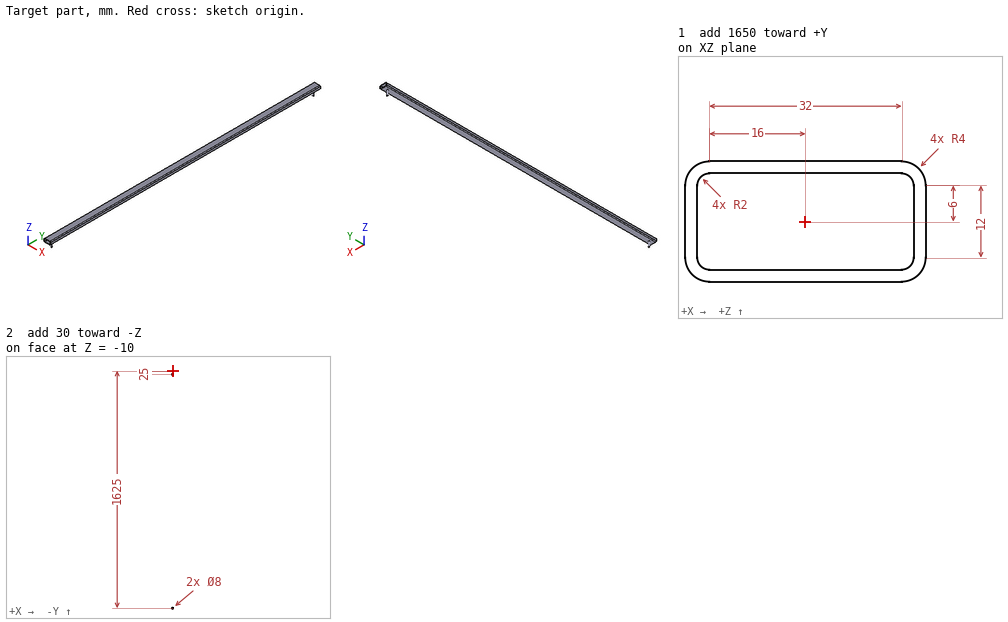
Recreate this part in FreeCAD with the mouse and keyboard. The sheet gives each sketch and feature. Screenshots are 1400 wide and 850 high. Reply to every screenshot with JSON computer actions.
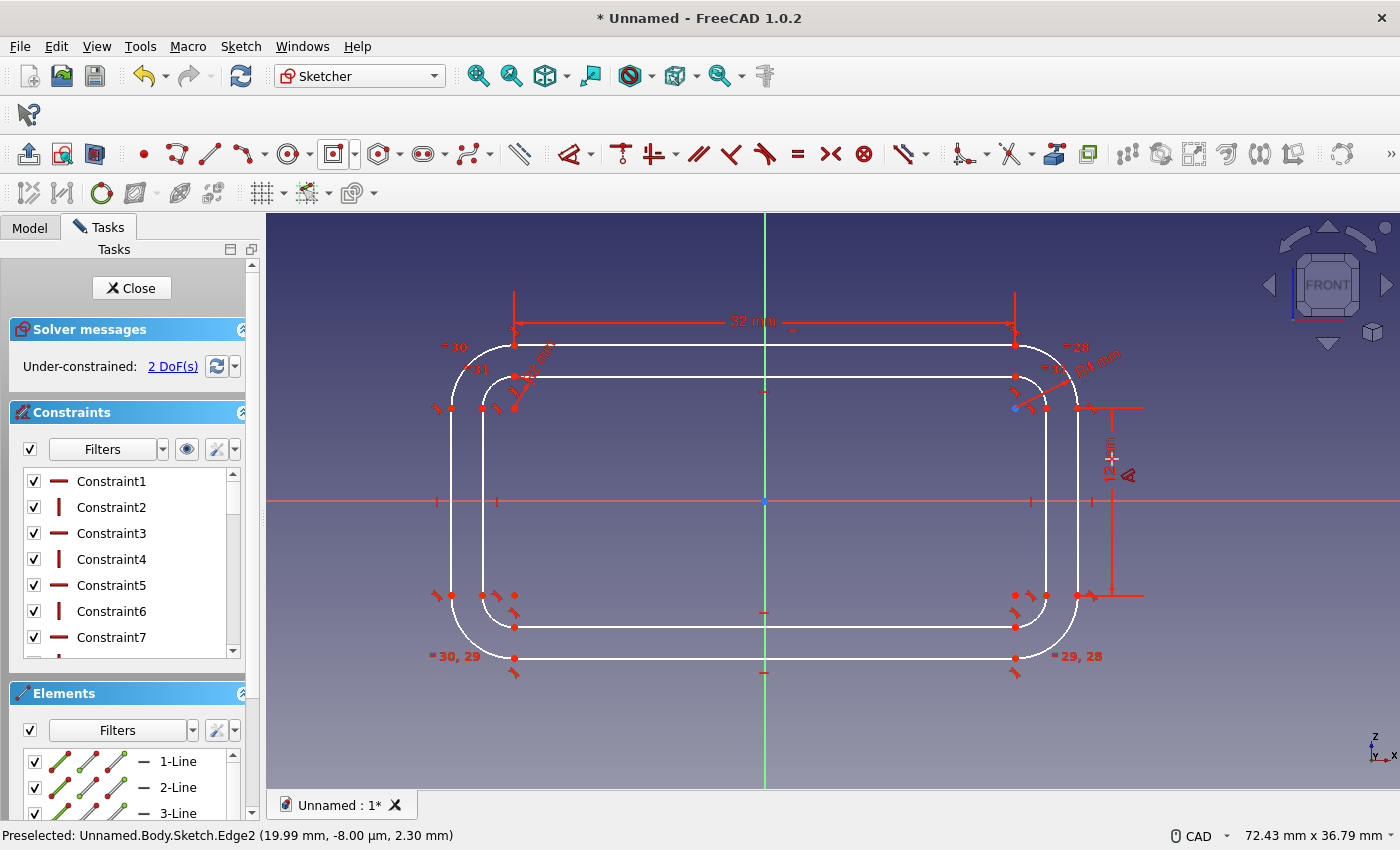
{"action": "left_click", "coordinate": [1078, 408]}
{"action": "left_click", "coordinate": [1112, 433]}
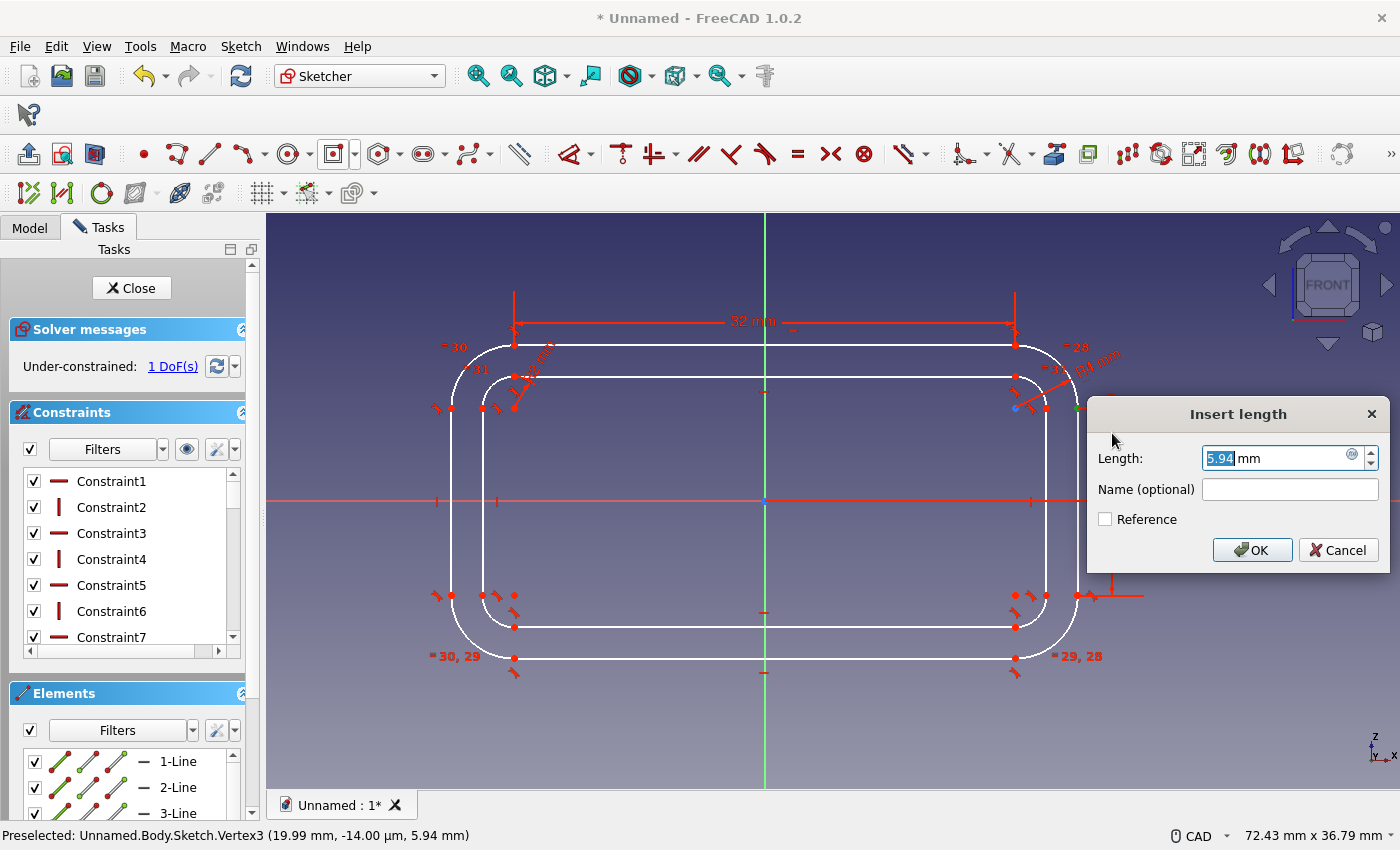
{"action": "type", "text": "6"}
{"action": "key", "text": "Return"}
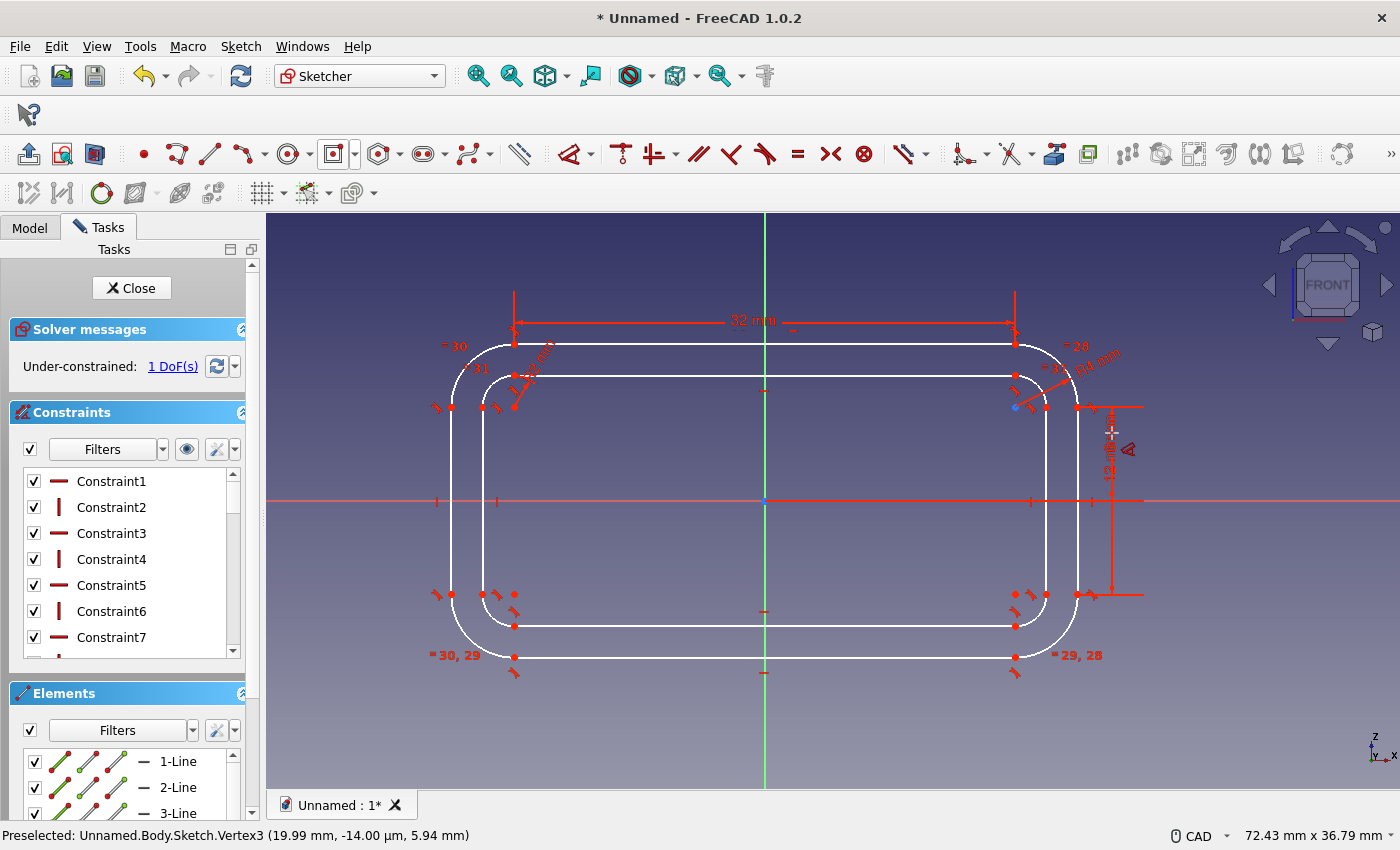
{"action": "left_click", "coordinate": [514, 344]}
{"action": "left_click", "coordinate": [639, 310]}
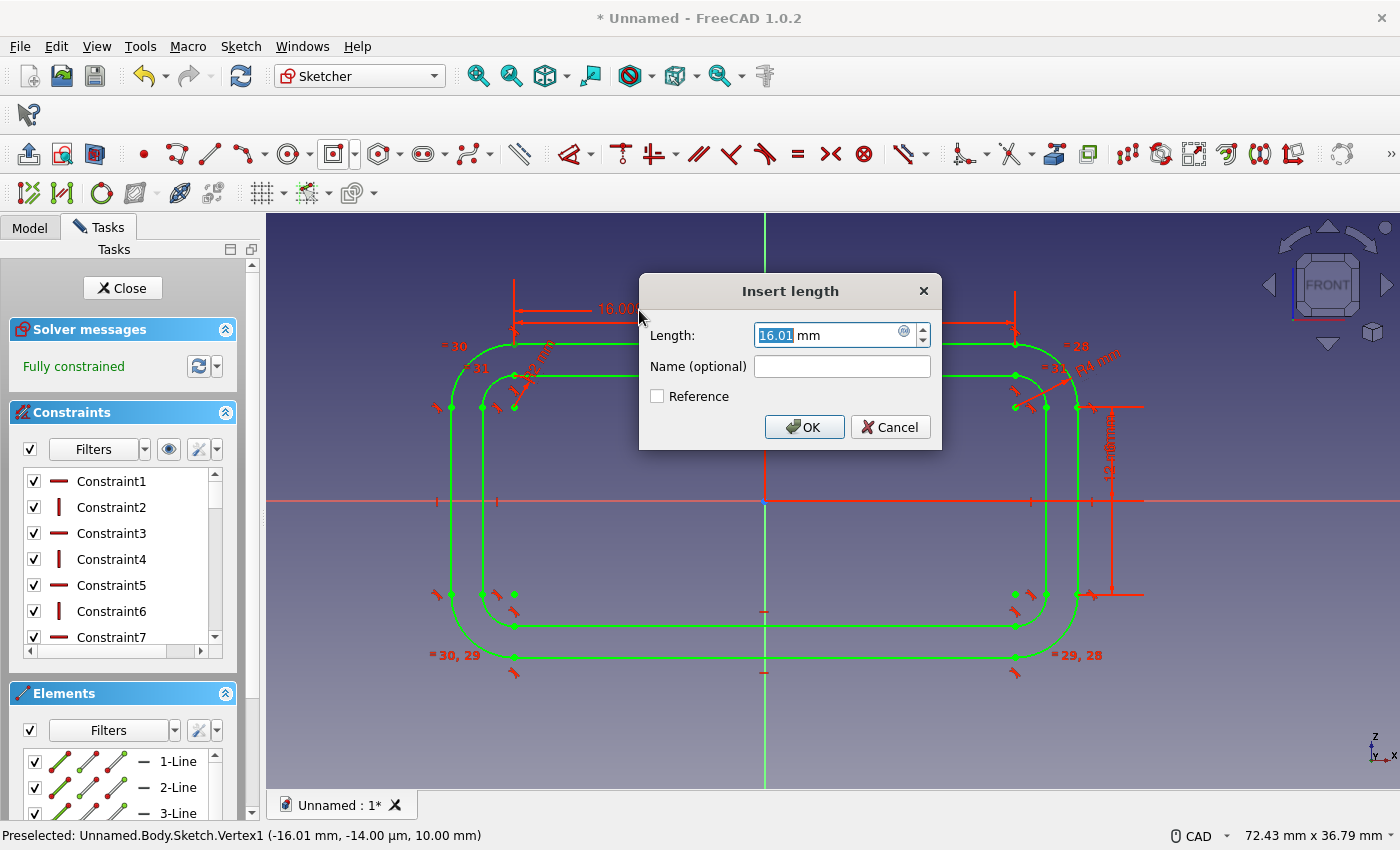
{"action": "type", "text": "16"}
{"action": "key", "text": "Return"}
{"action": "key", "text": "Escape"}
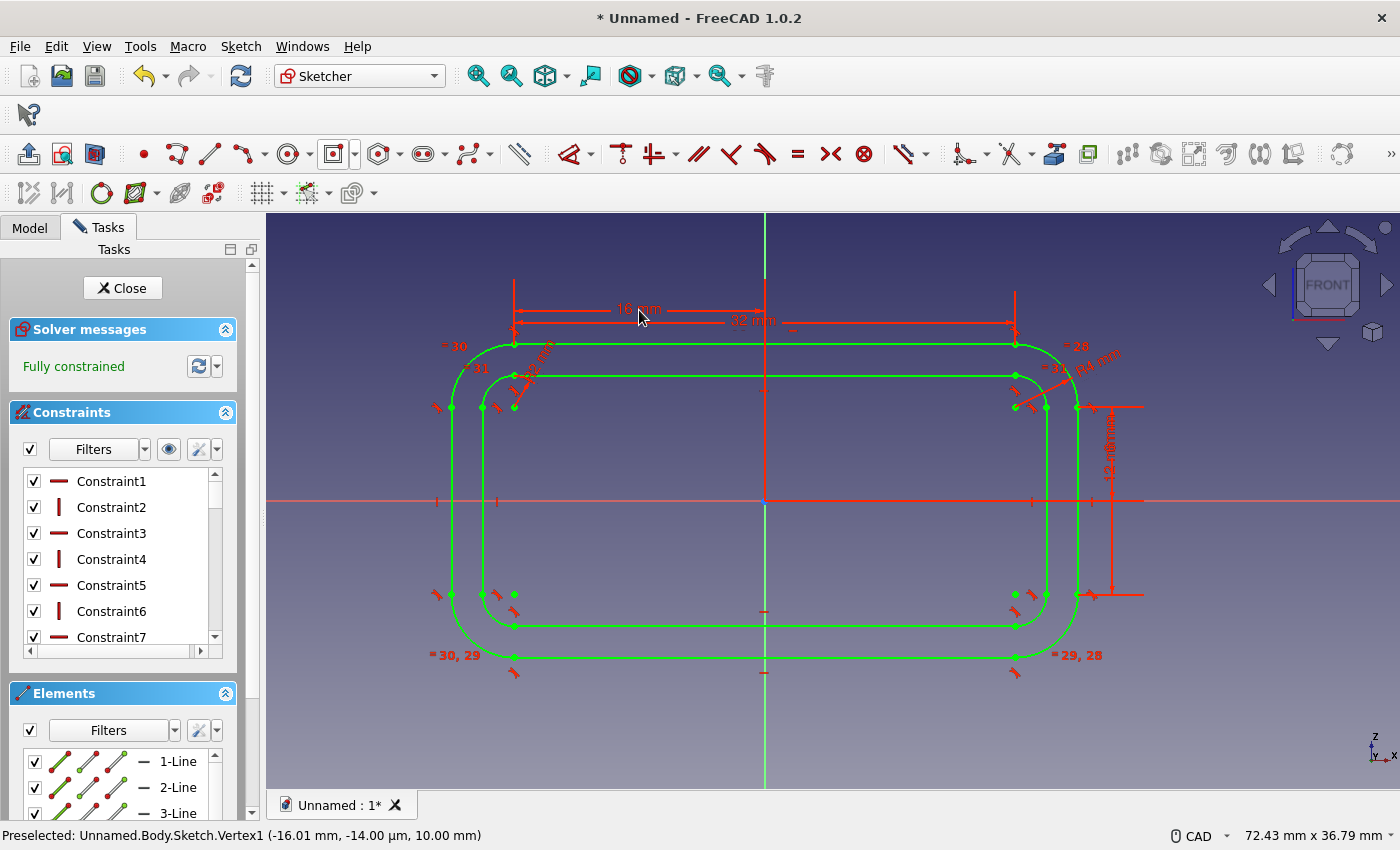
{"action": "left_click", "coordinate": [123, 288]}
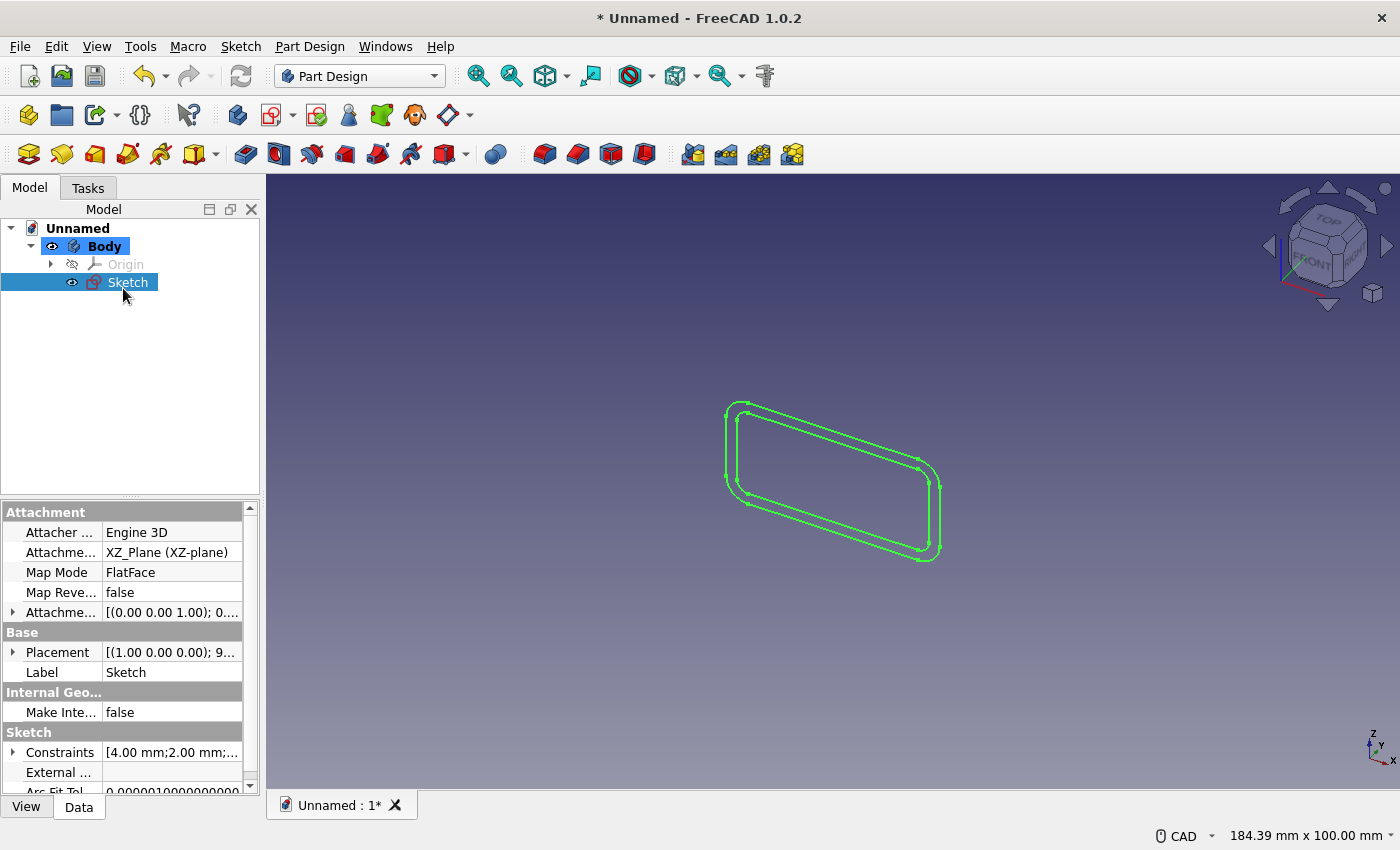
{"action": "left_click", "coordinate": [29, 154]}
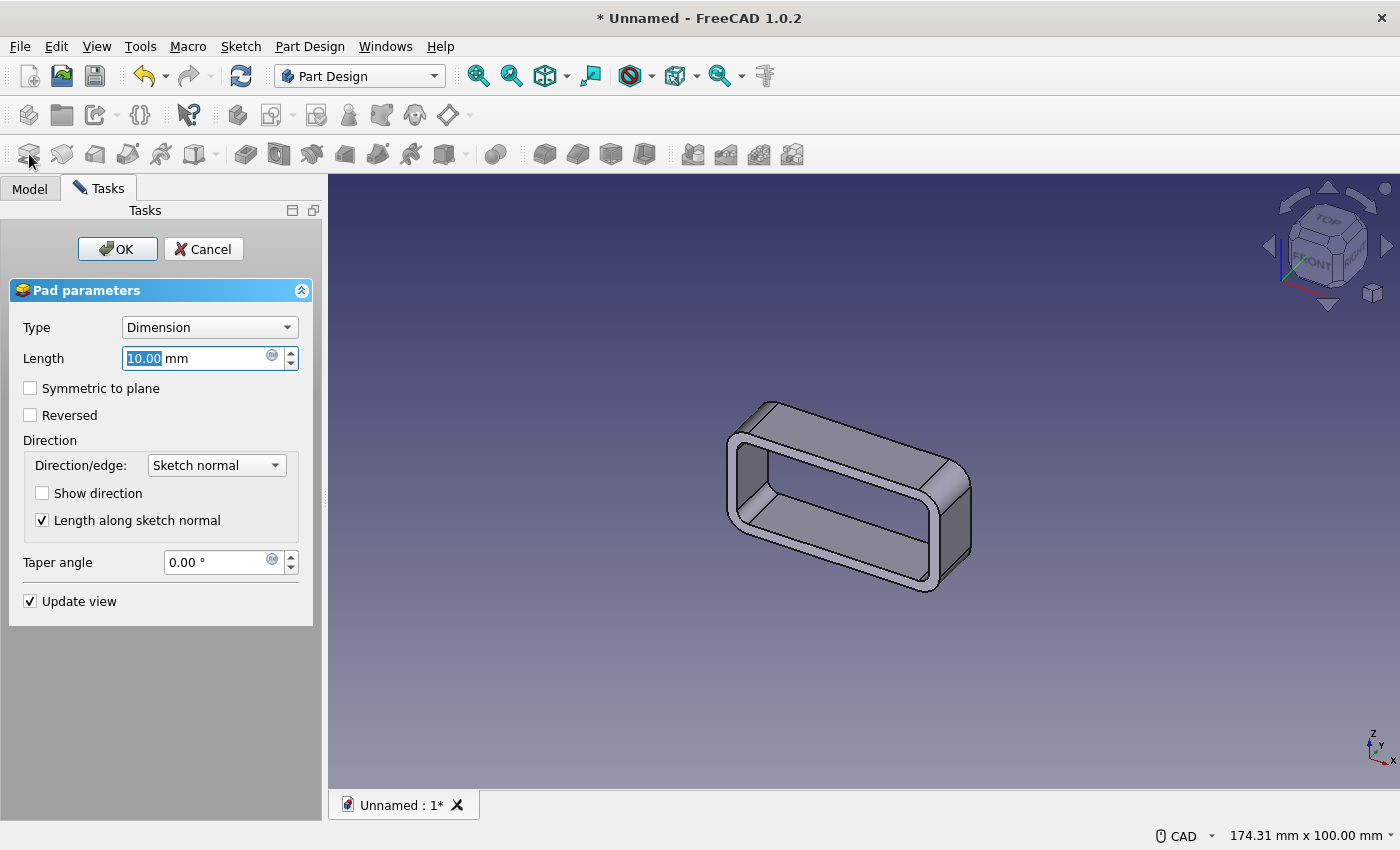
{"action": "type", "text": "1650"}
{"action": "key", "text": "Tab"}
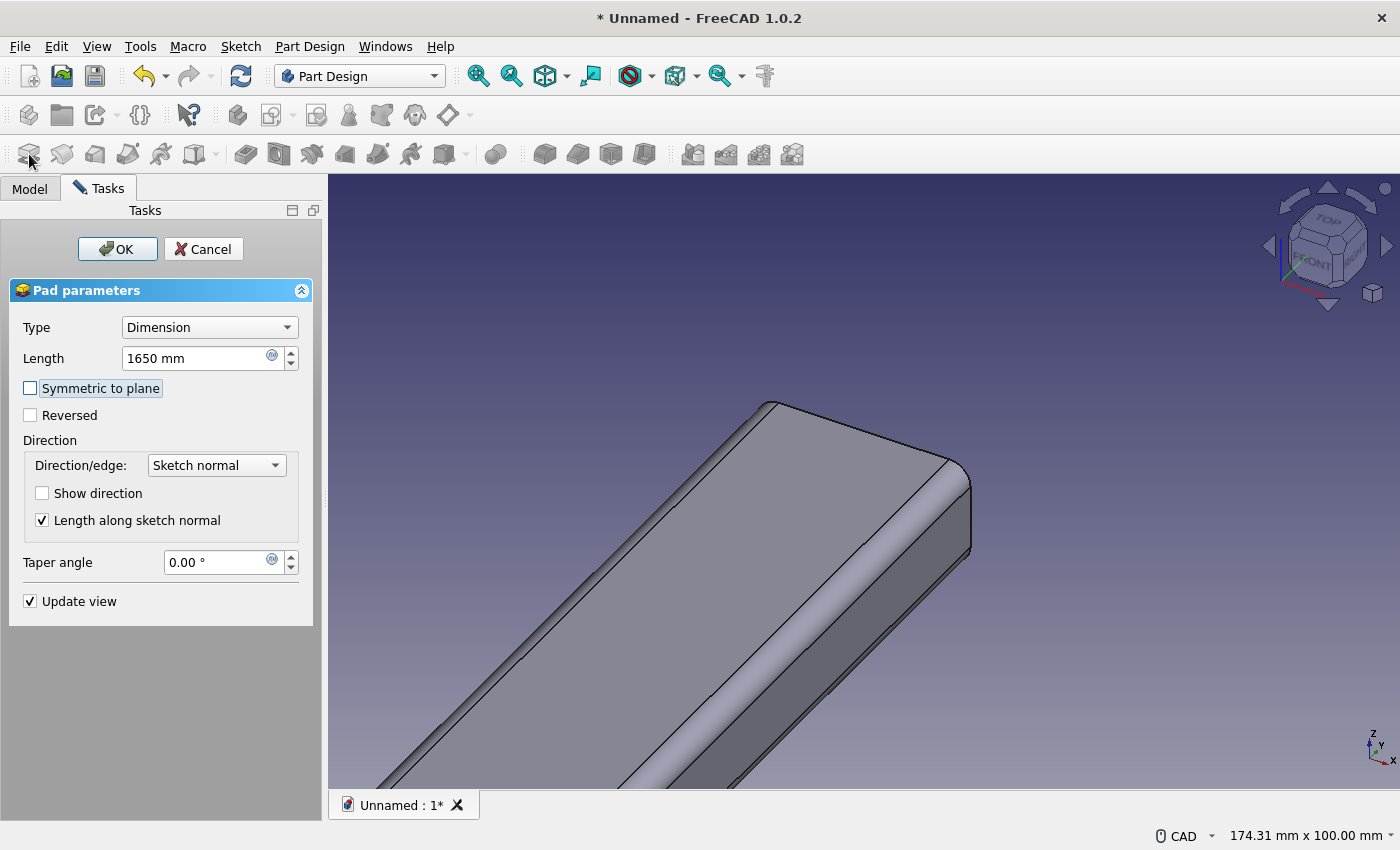
{"action": "left_click", "coordinate": [31, 415]}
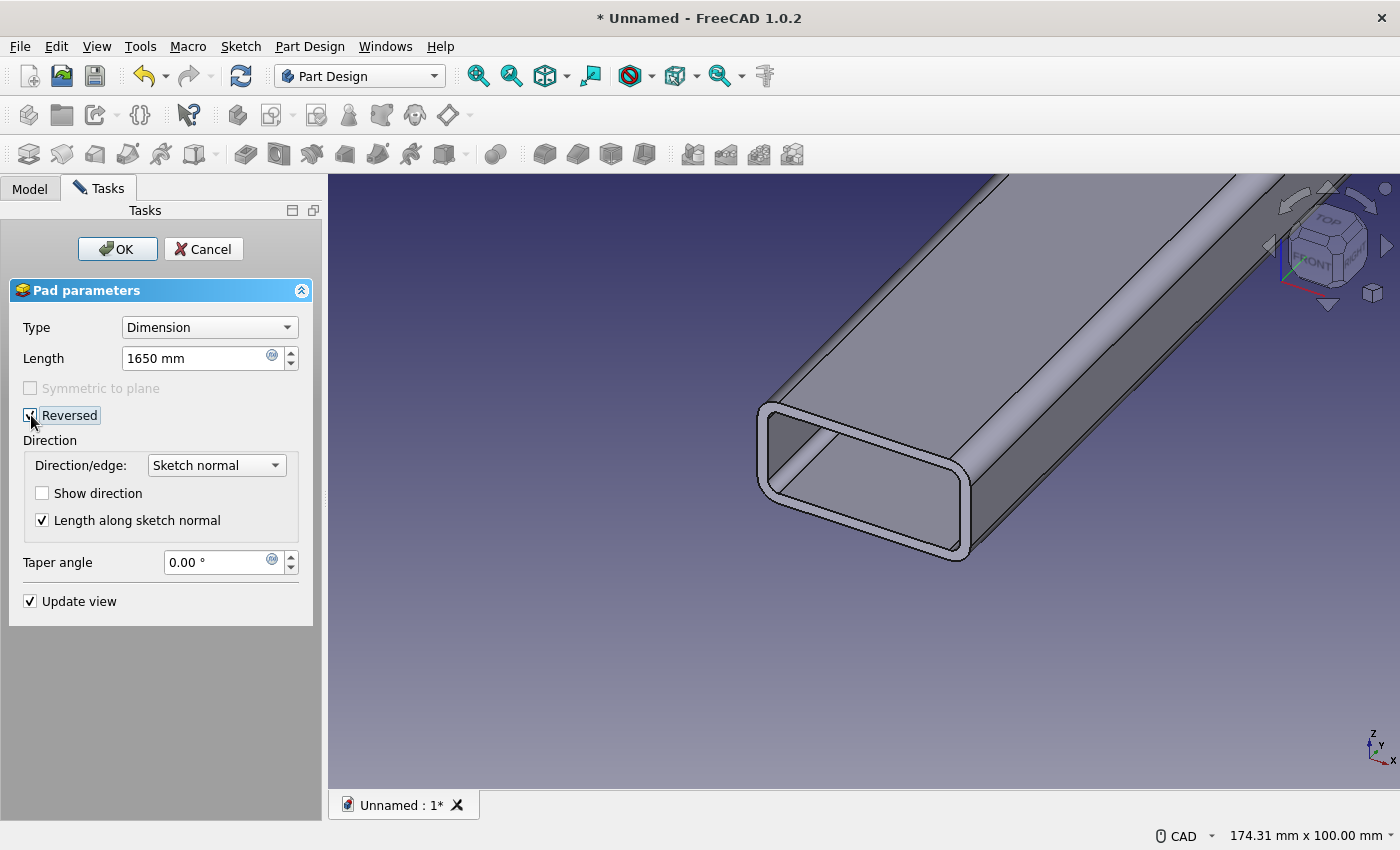
{"action": "left_click", "coordinate": [118, 249]}